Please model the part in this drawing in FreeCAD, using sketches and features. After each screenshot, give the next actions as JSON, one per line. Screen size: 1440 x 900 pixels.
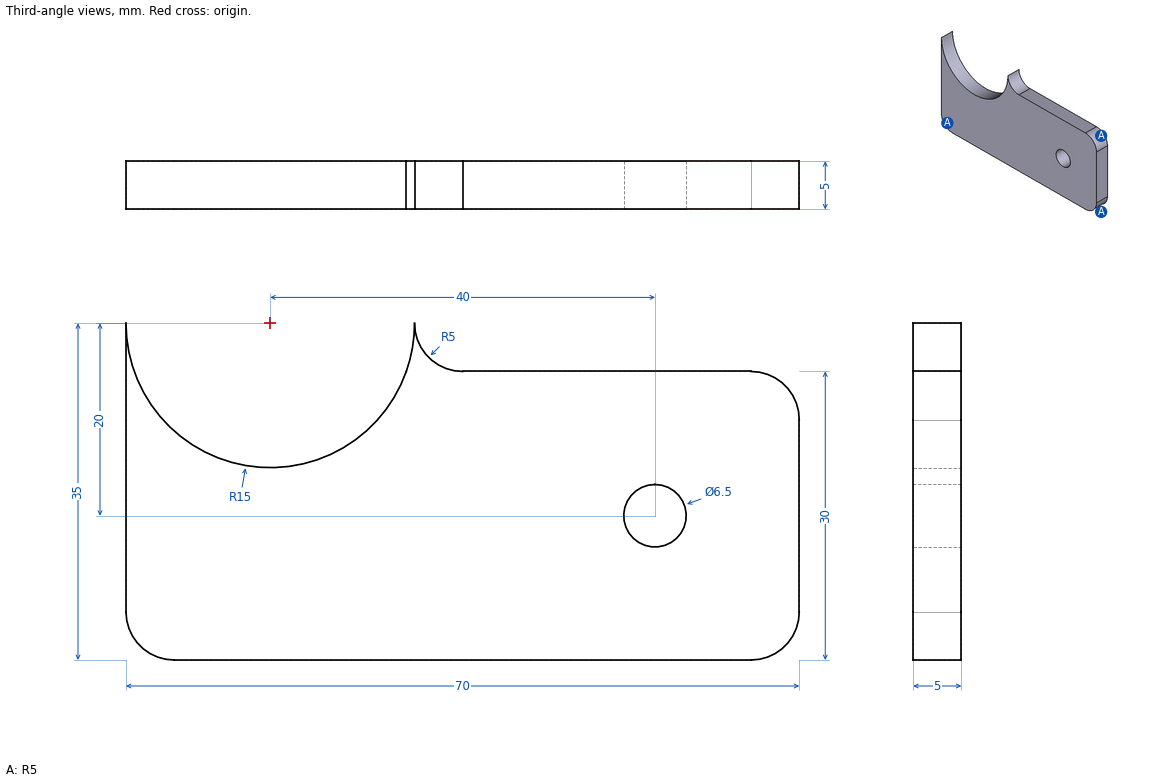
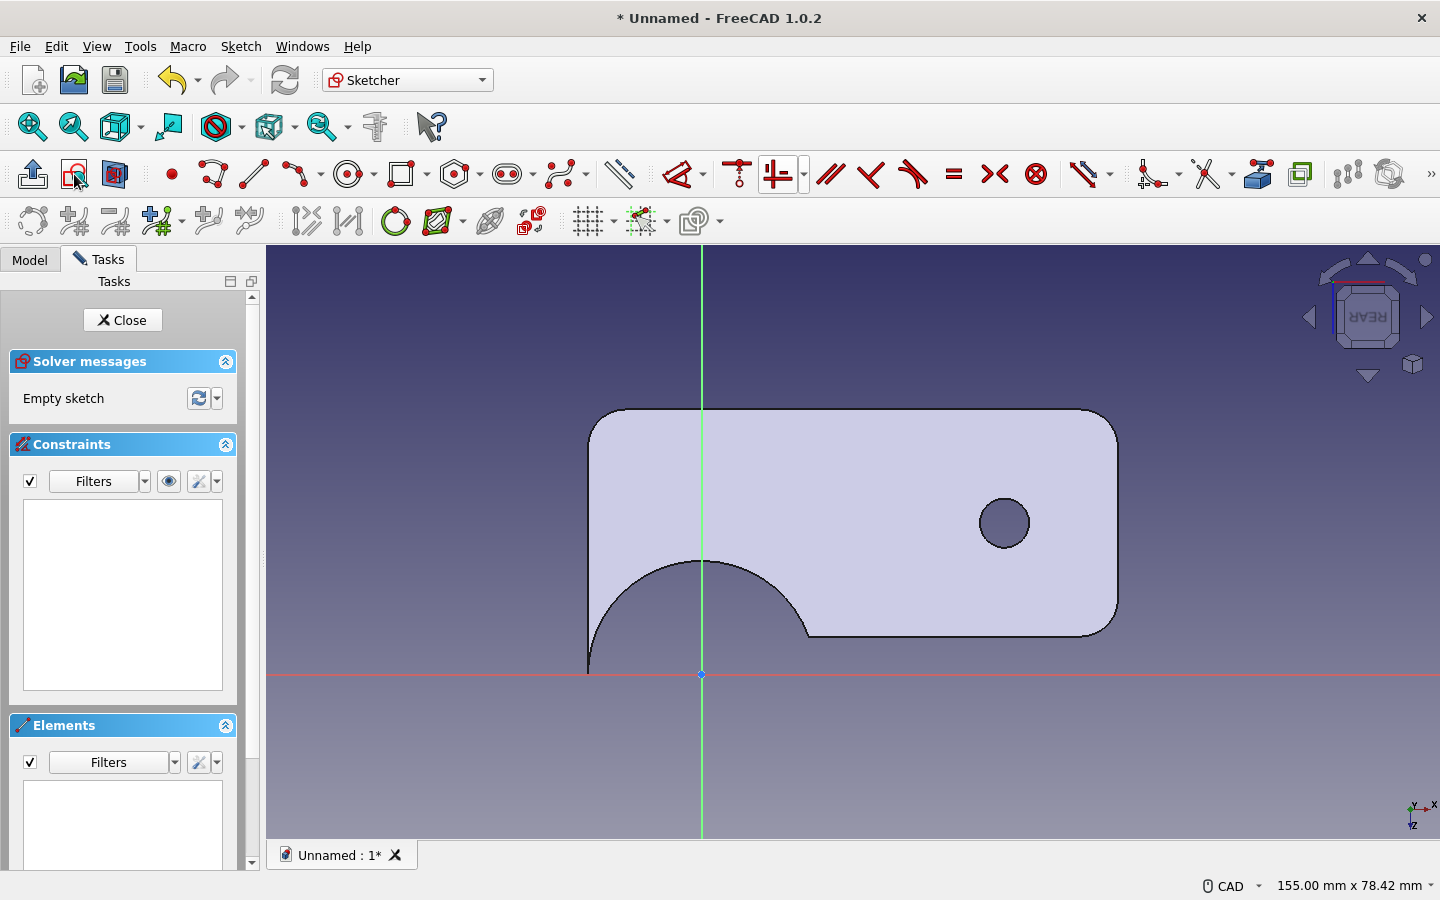
{"action": "scroll", "coordinate": [835, 667], "scroll_direction": "up", "scroll_amount": 12}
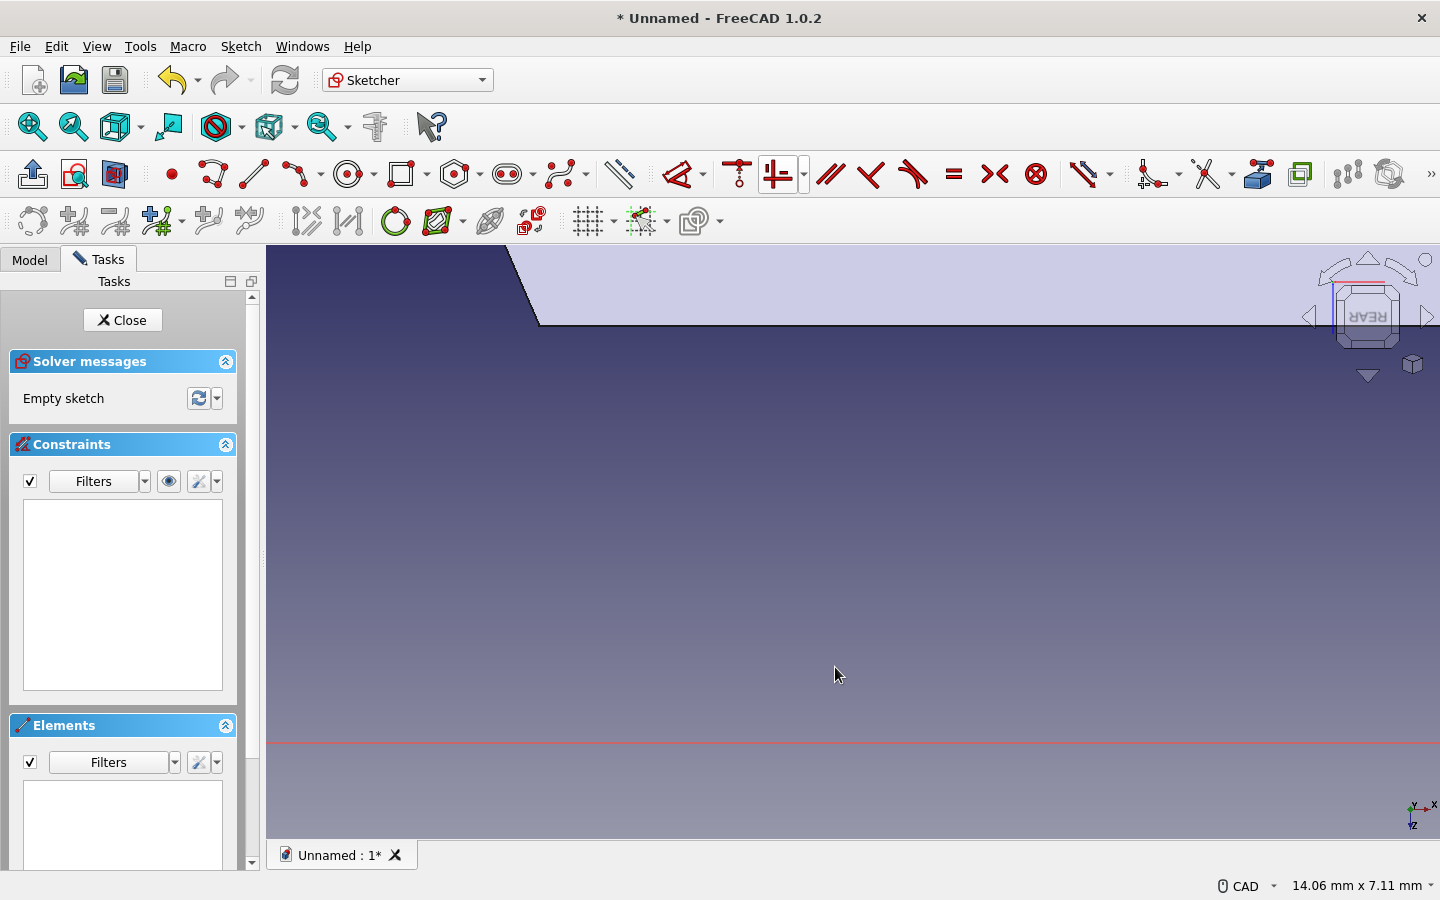
{"action": "left_click", "coordinate": [254, 174]}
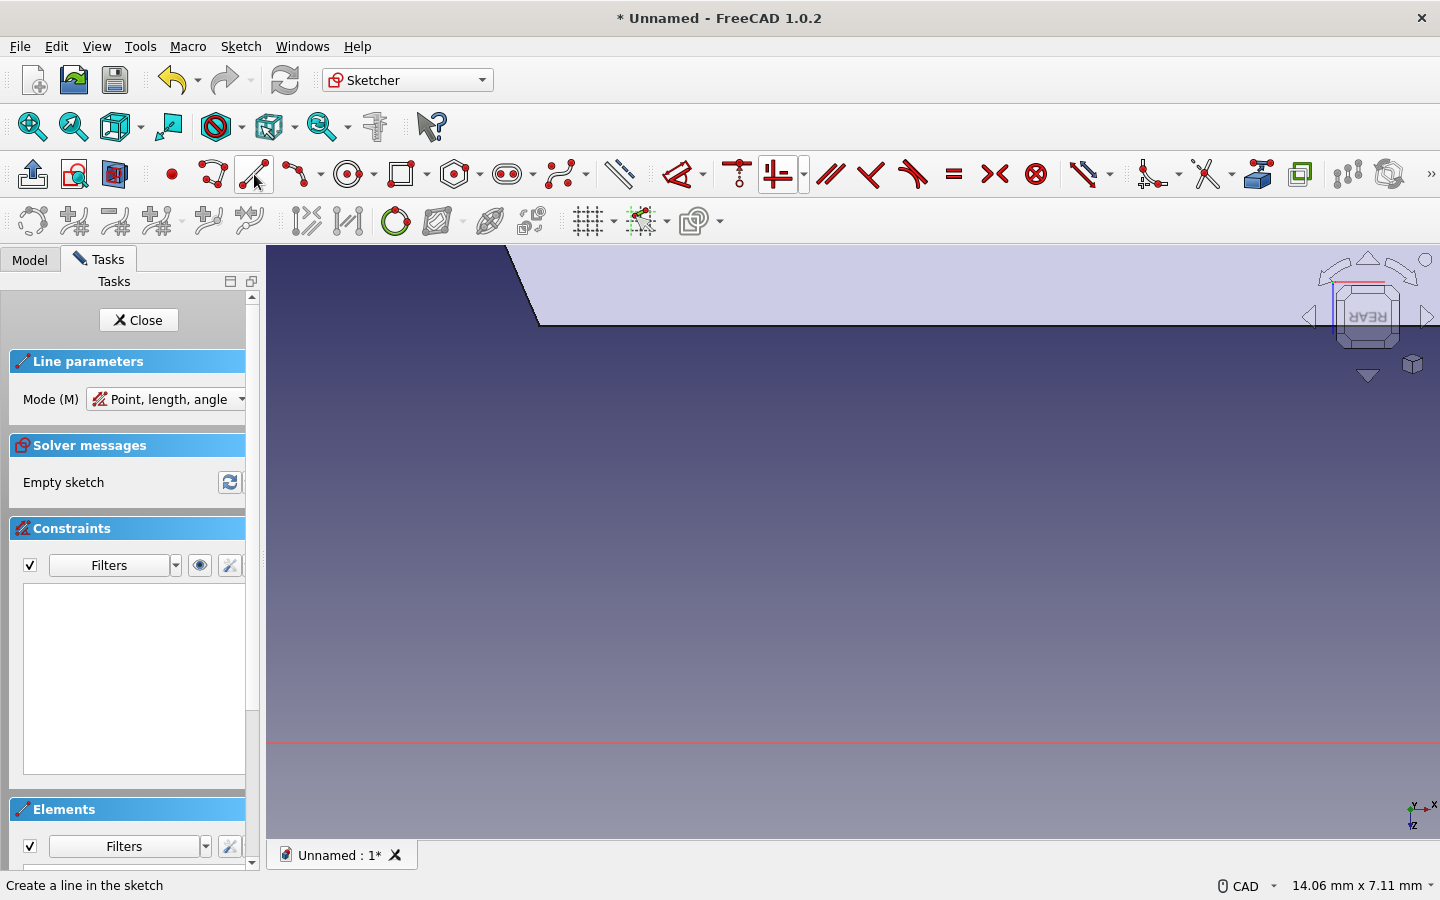
{"action": "left_click", "coordinate": [1029, 326]}
{"action": "left_click", "coordinate": [539, 326]}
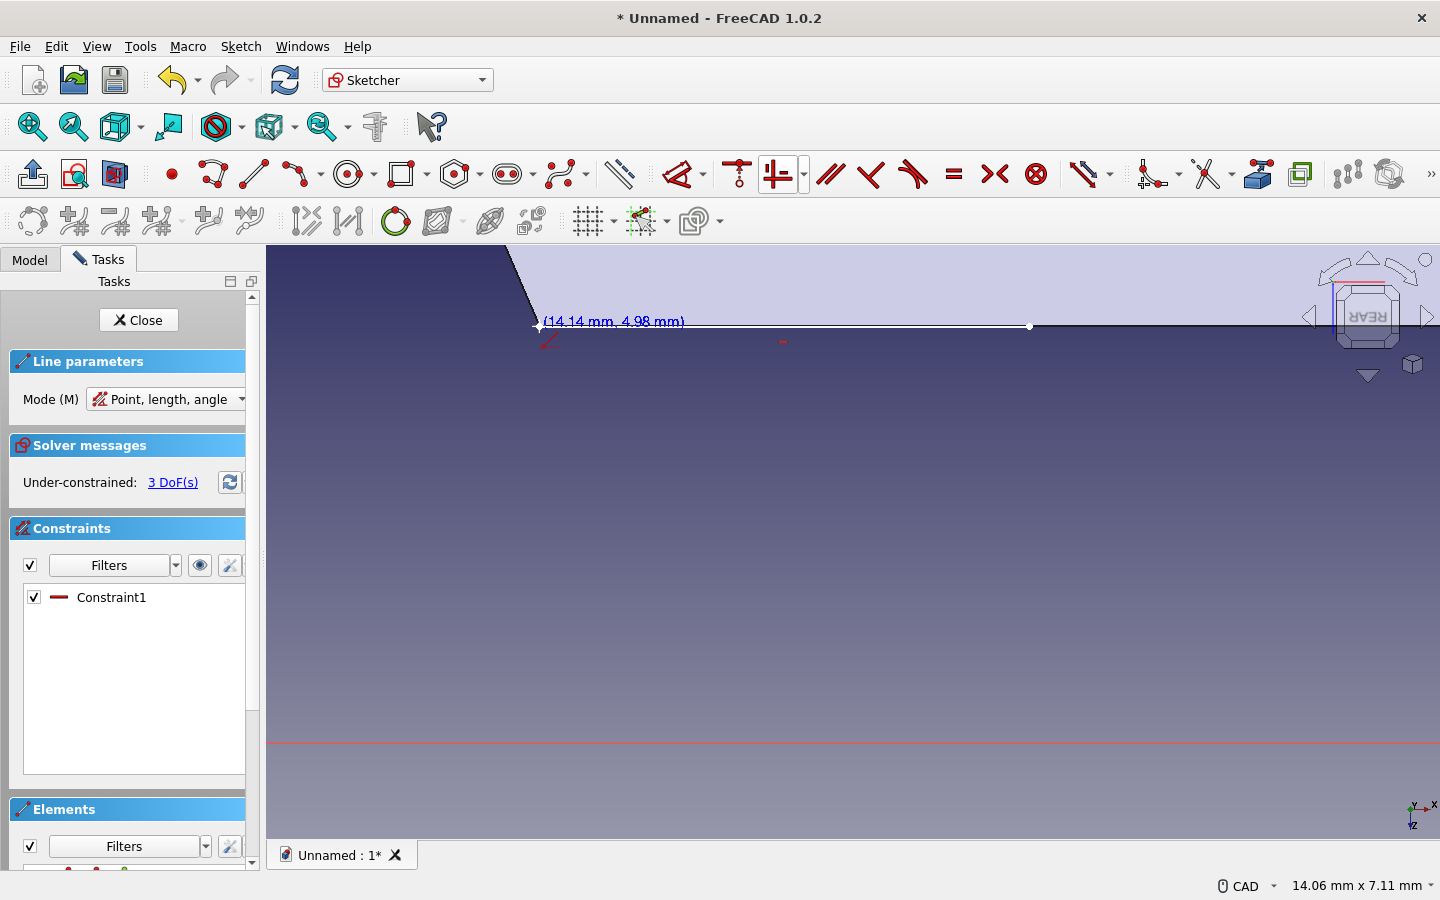
{"action": "left_click", "coordinate": [294, 174]}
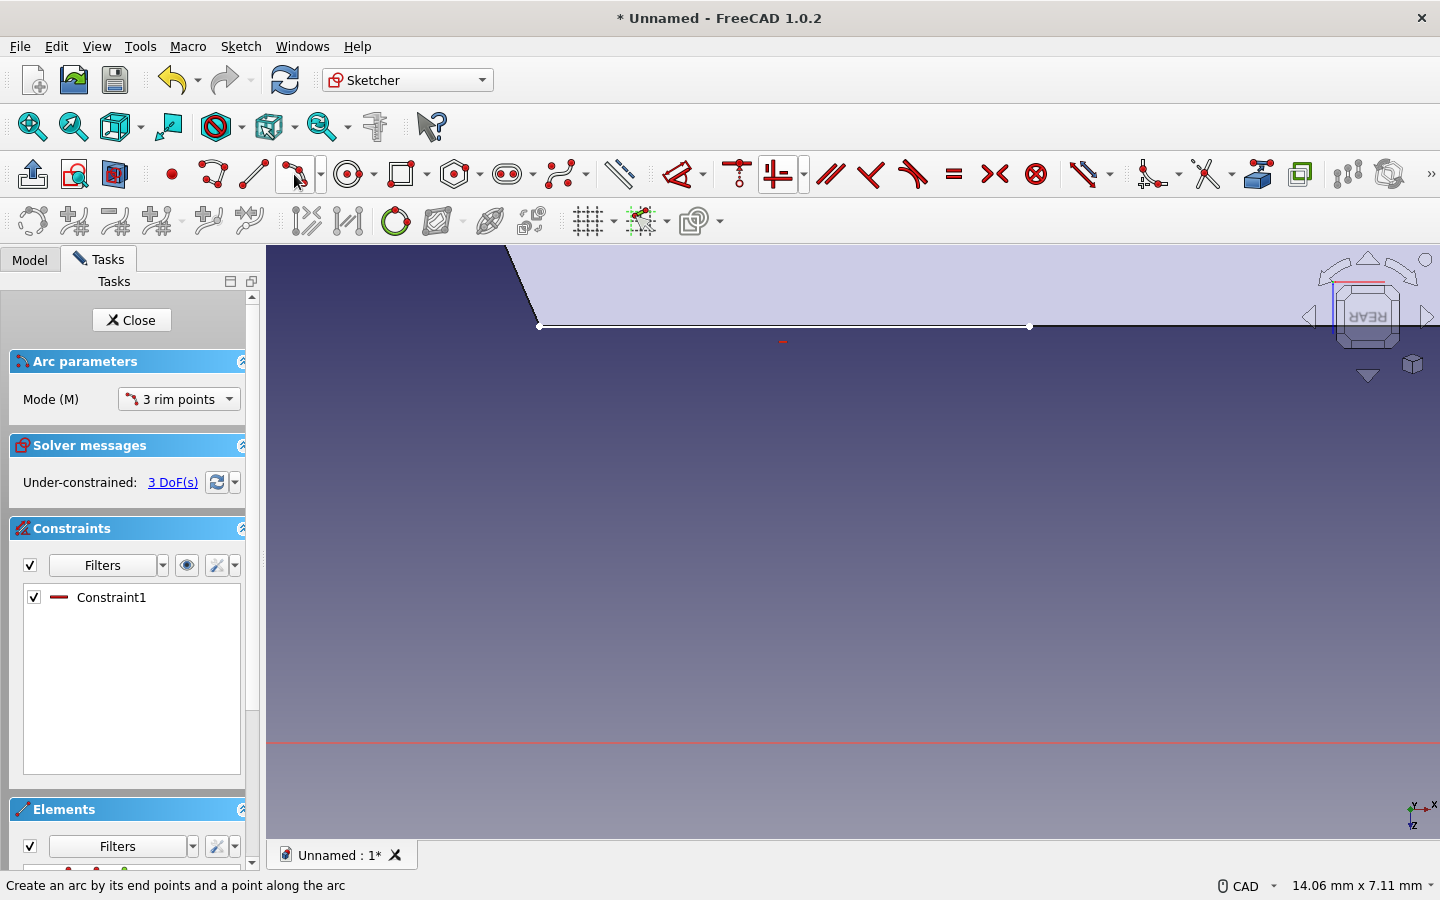
{"action": "left_click", "coordinate": [539, 327]}
{"action": "left_click", "coordinate": [611, 743]}
{"action": "left_click", "coordinate": [593, 531]}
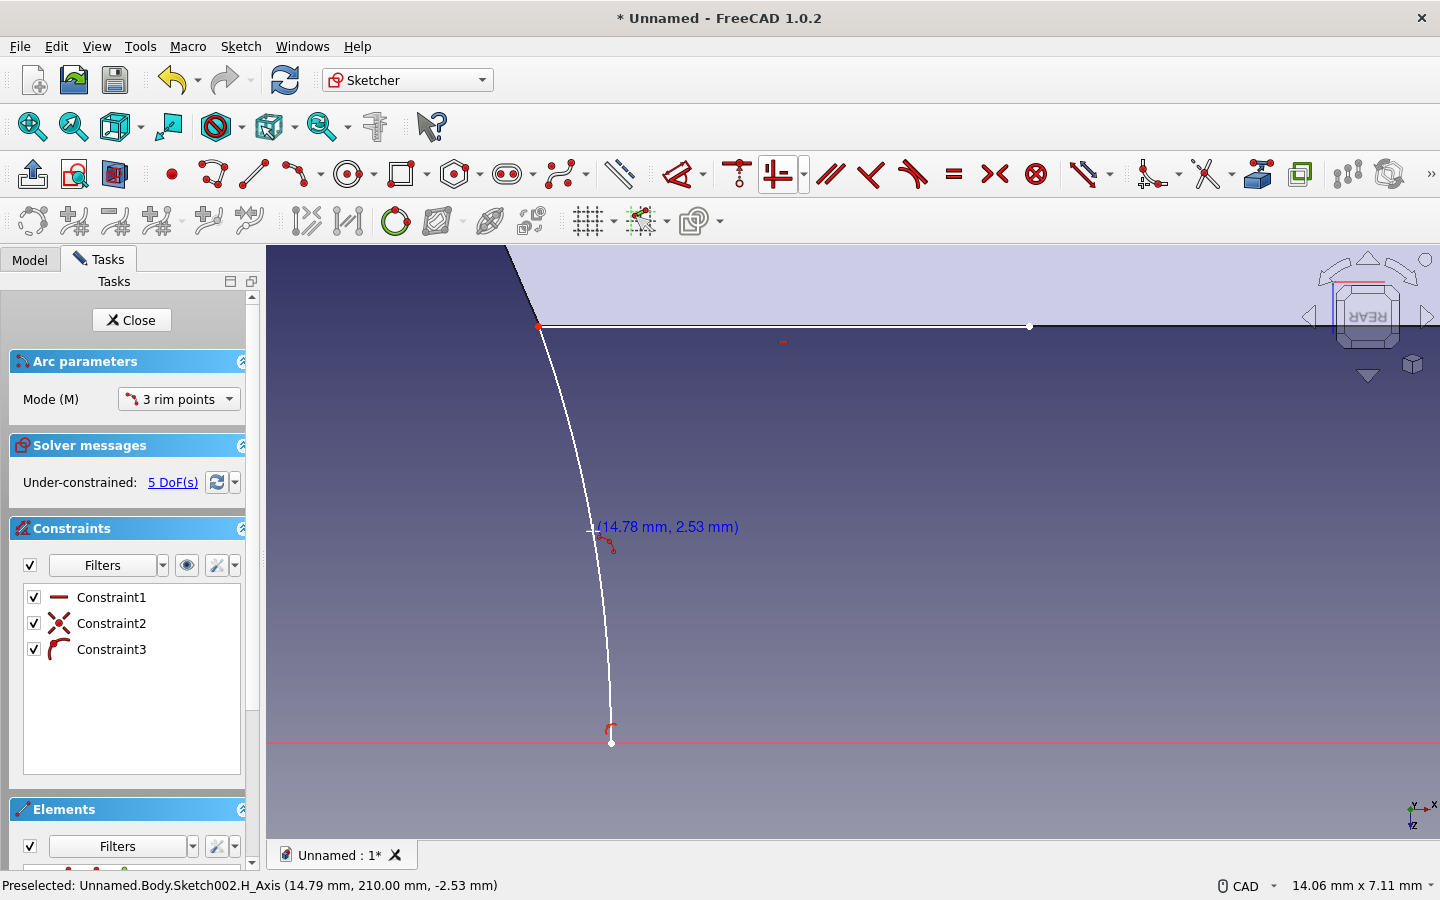
{"action": "left_click", "coordinate": [611, 743]}
{"action": "left_click", "coordinate": [1029, 327]}
{"action": "left_click", "coordinate": [733, 448]}
{"action": "key", "text": "Escape"}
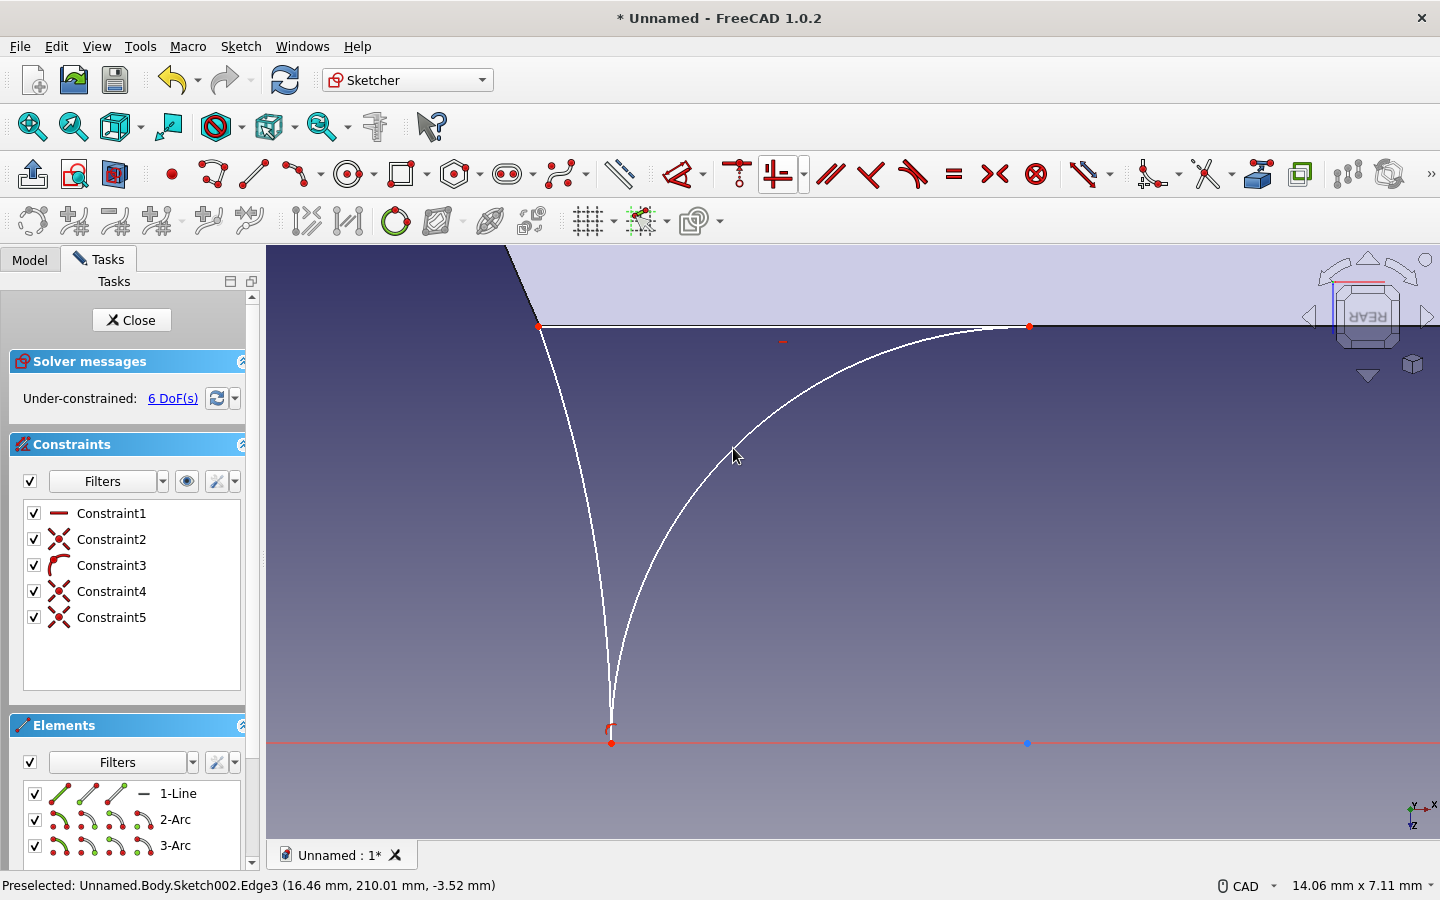
{"action": "left_click", "coordinate": [882, 327]}